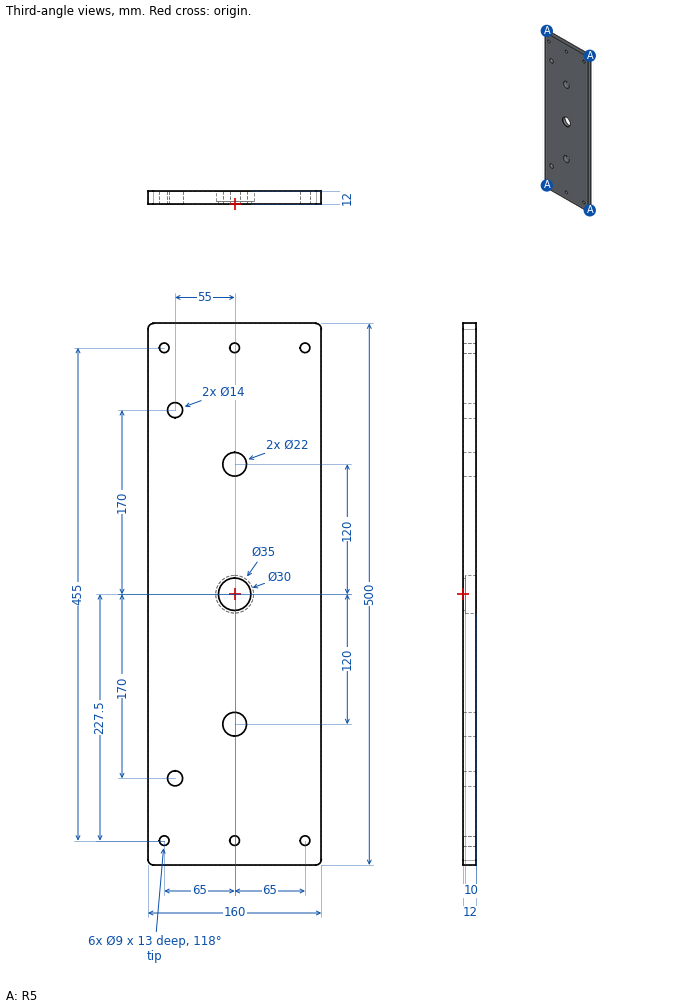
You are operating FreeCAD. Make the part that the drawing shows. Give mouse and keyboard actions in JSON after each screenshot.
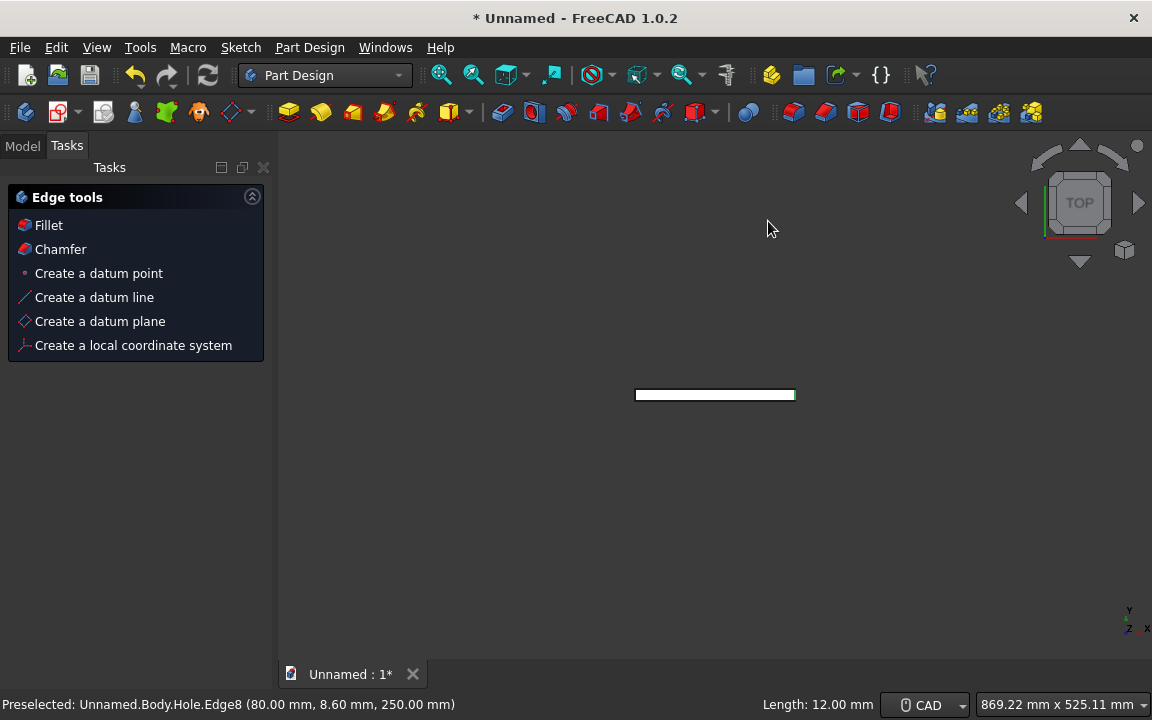
{"action": "left_click", "coordinate": [635, 394], "text": "ctrl"}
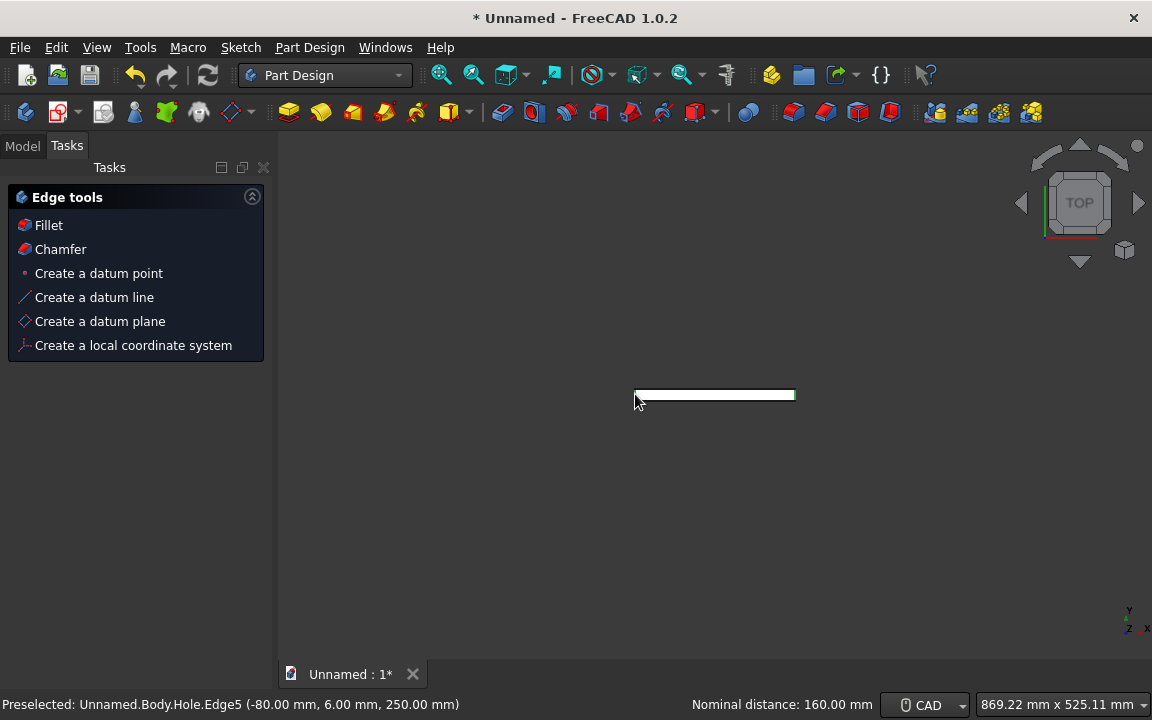
{"action": "scroll", "coordinate": [635, 394], "scroll_direction": "up", "scroll_amount": 6}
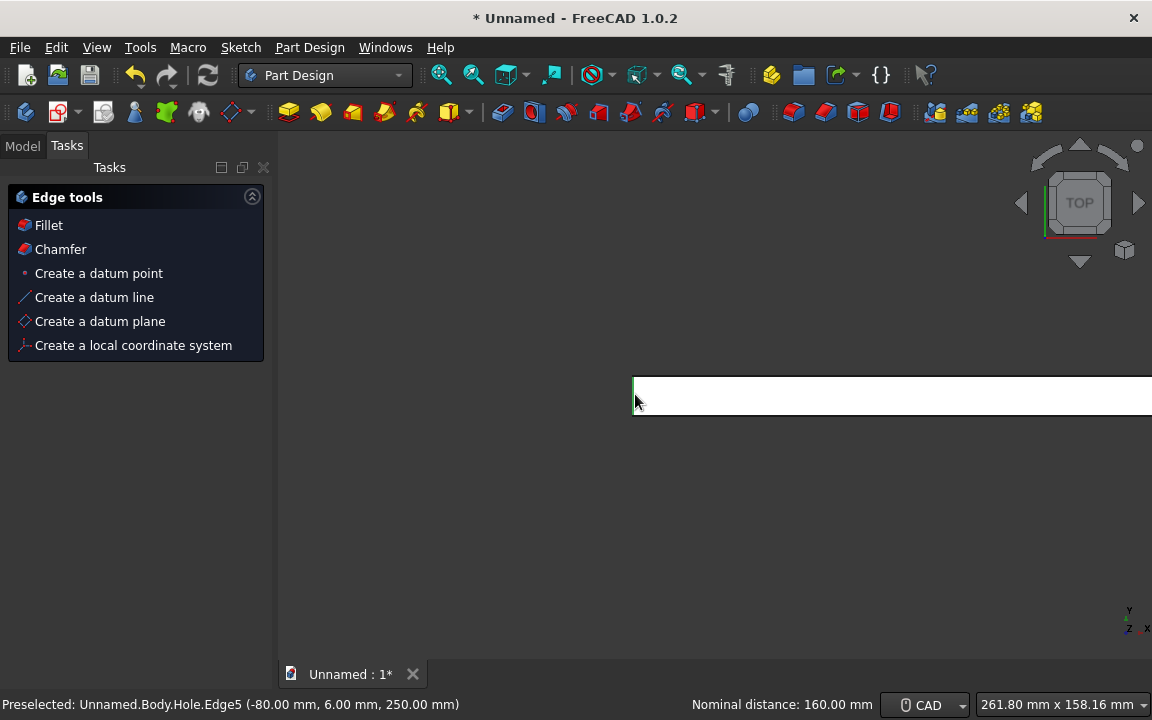
{"action": "key", "text": "v f"}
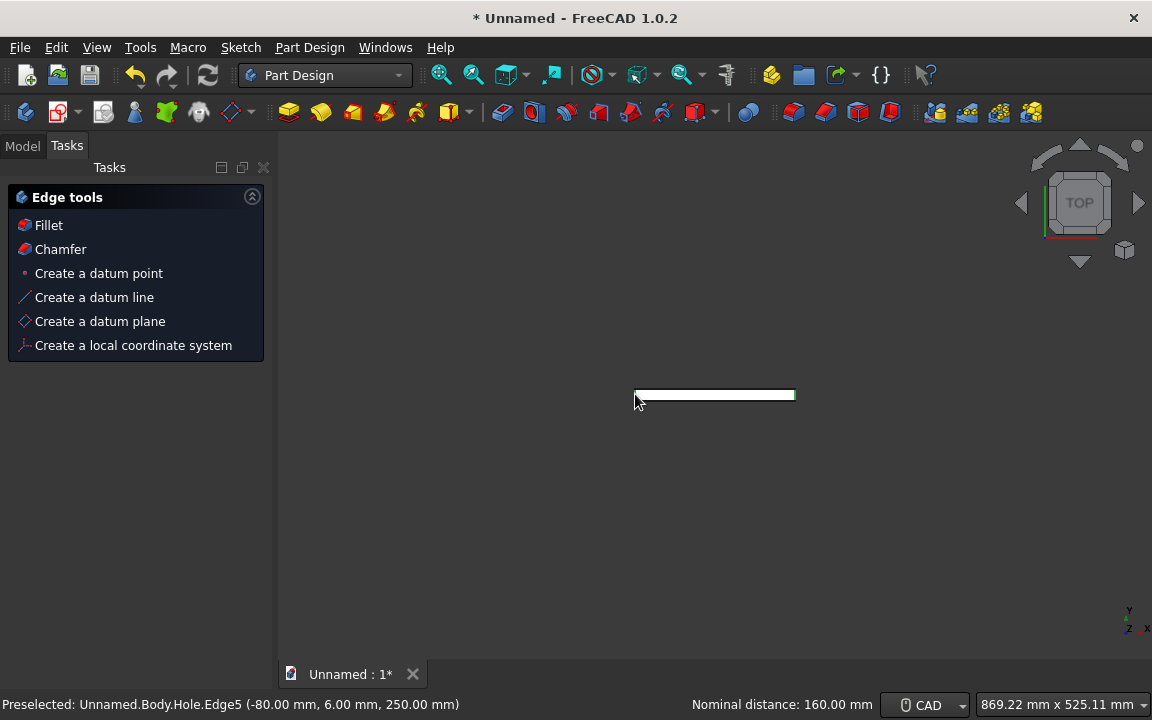
{"action": "key", "text": "1"}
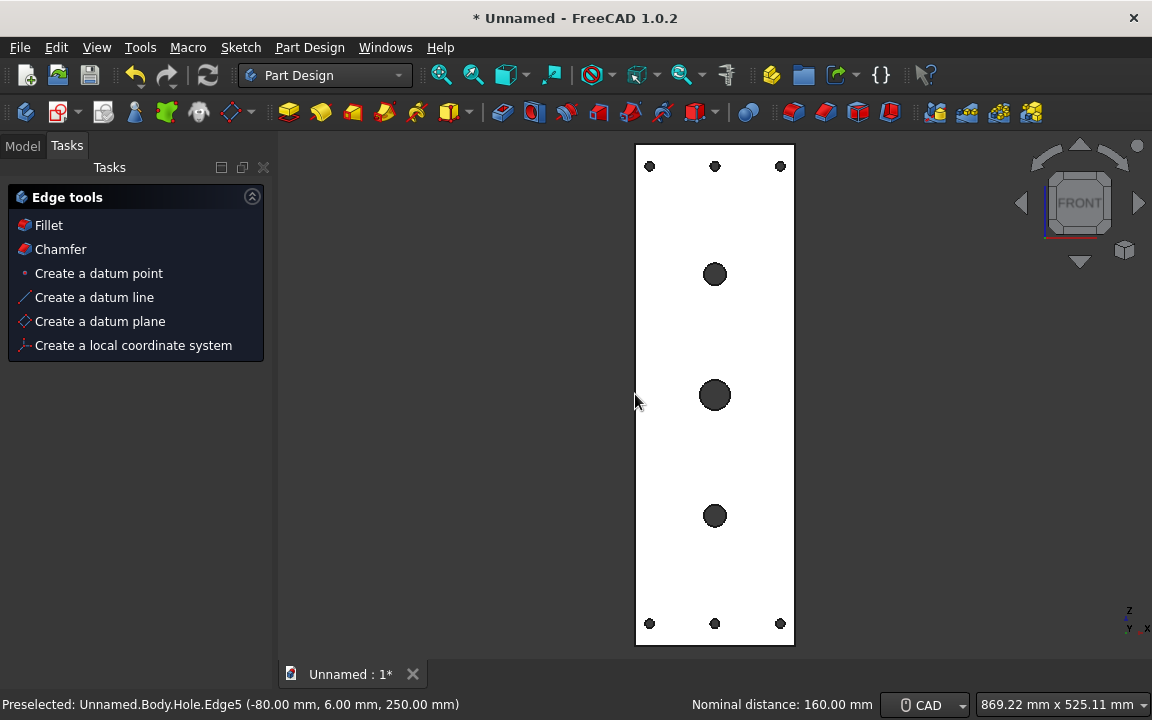
{"action": "key", "text": "3"}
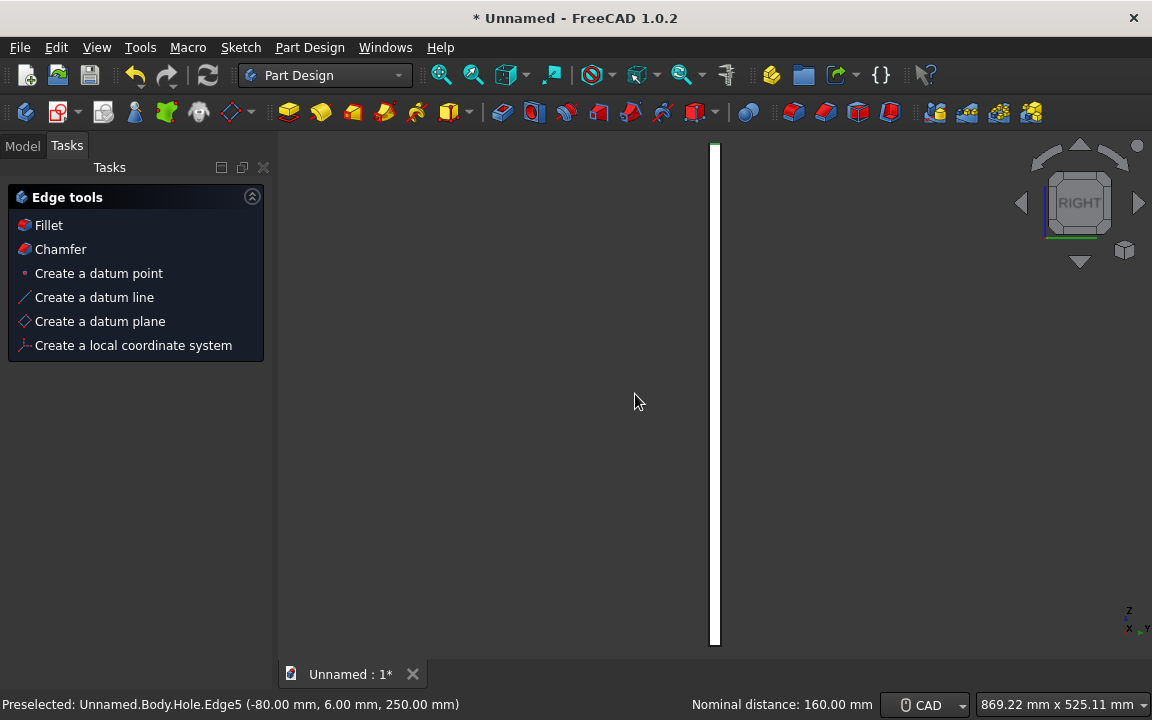
{"action": "key", "text": "5"}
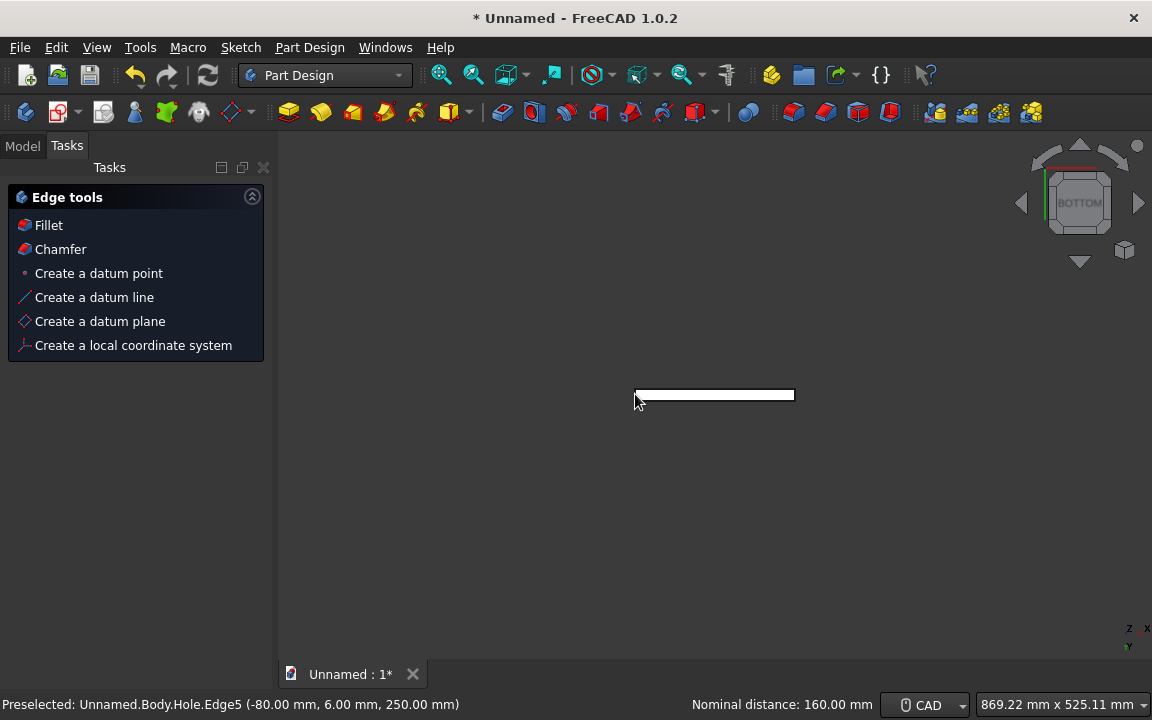
{"action": "left_click", "coordinate": [442, 76]}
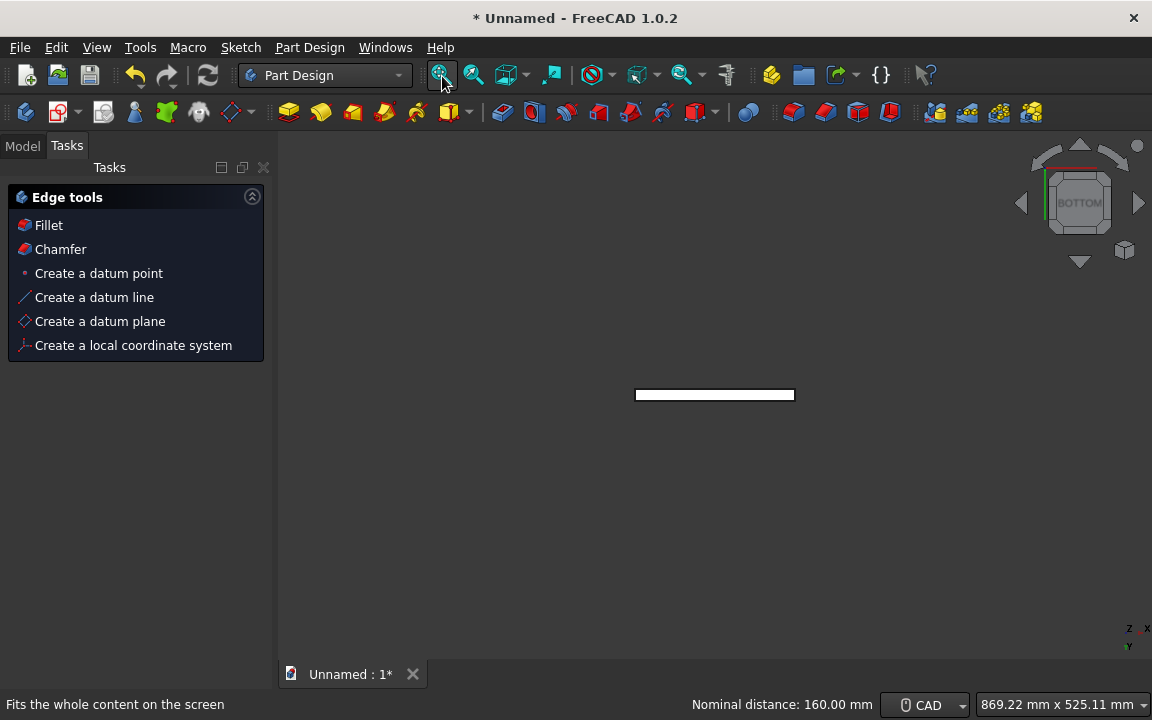
{"action": "left_click", "coordinate": [635, 394], "text": "ctrl"}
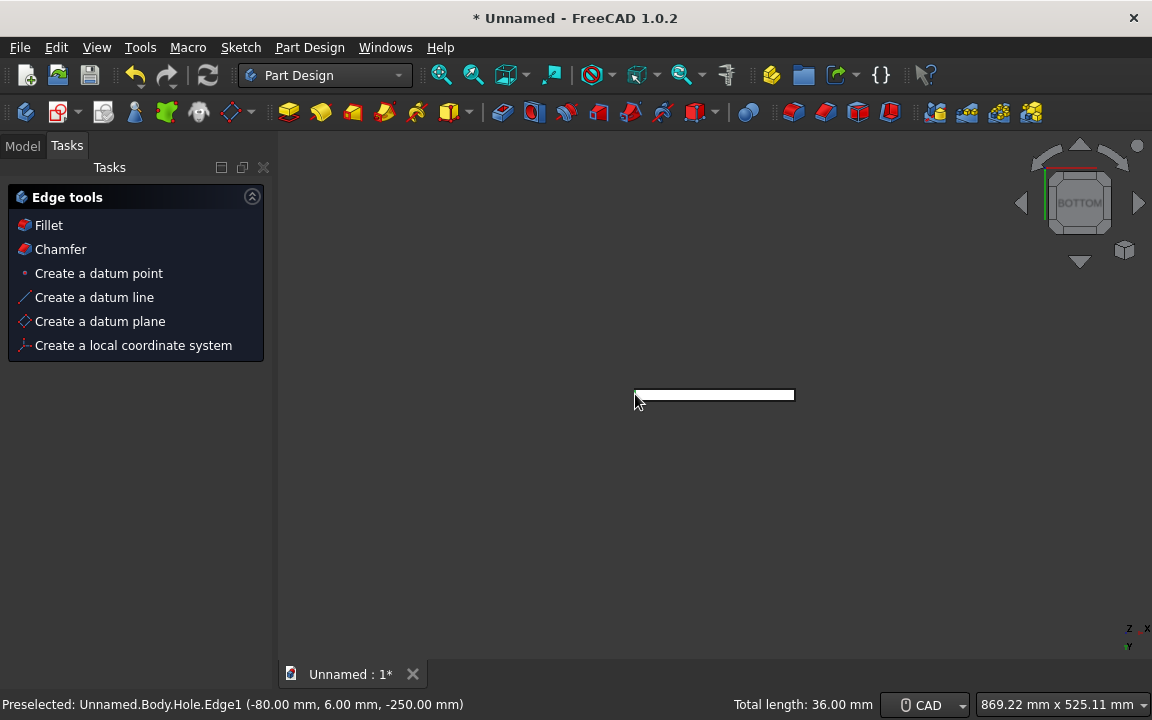
{"action": "left_click", "coordinate": [795, 394], "text": "ctrl"}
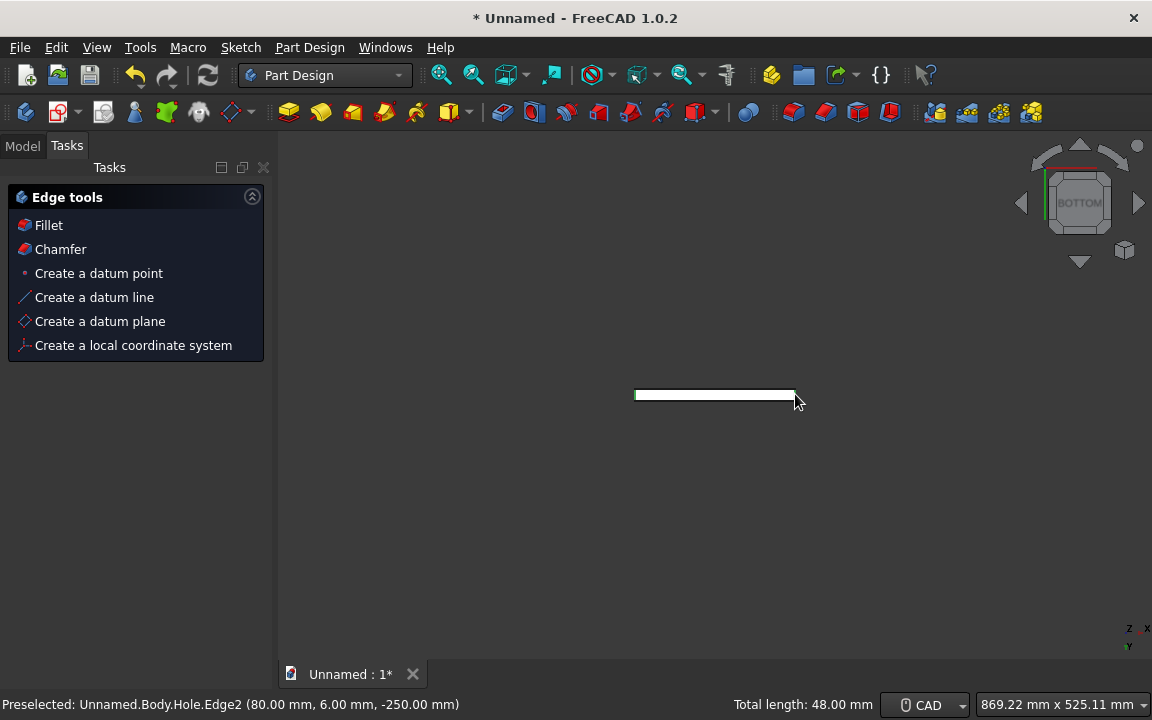
{"action": "left_click", "coordinate": [794, 112]}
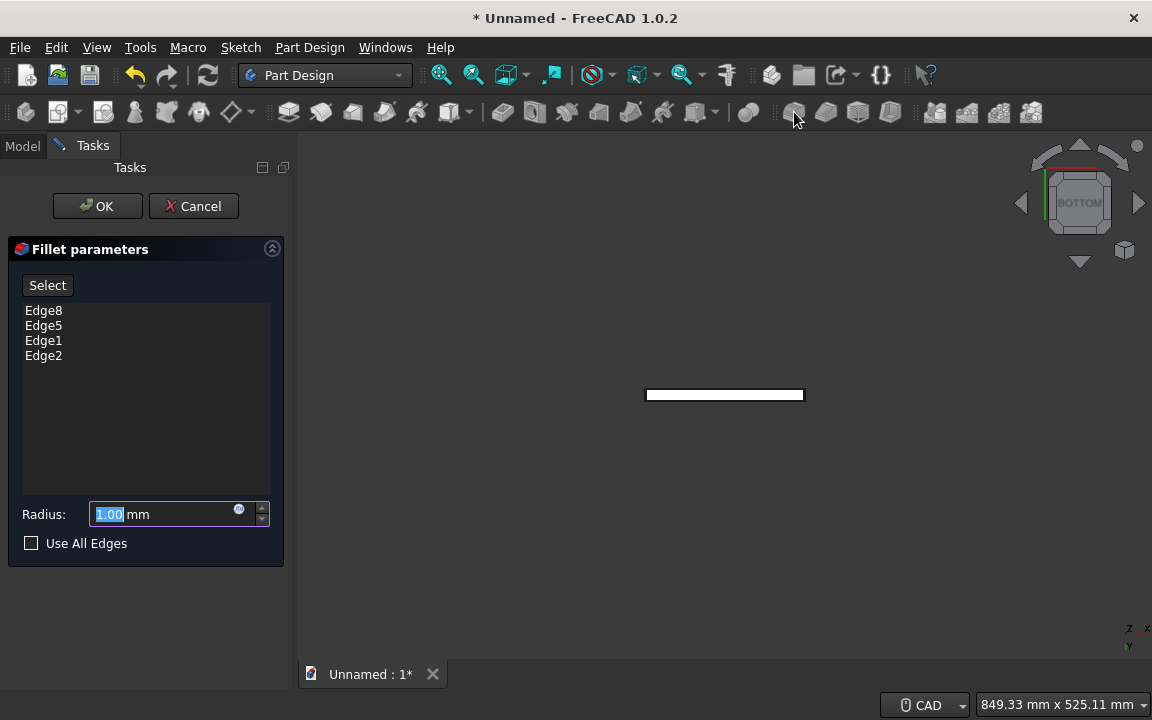
{"action": "type", "text": "5"}
{"action": "key", "text": "Tab"}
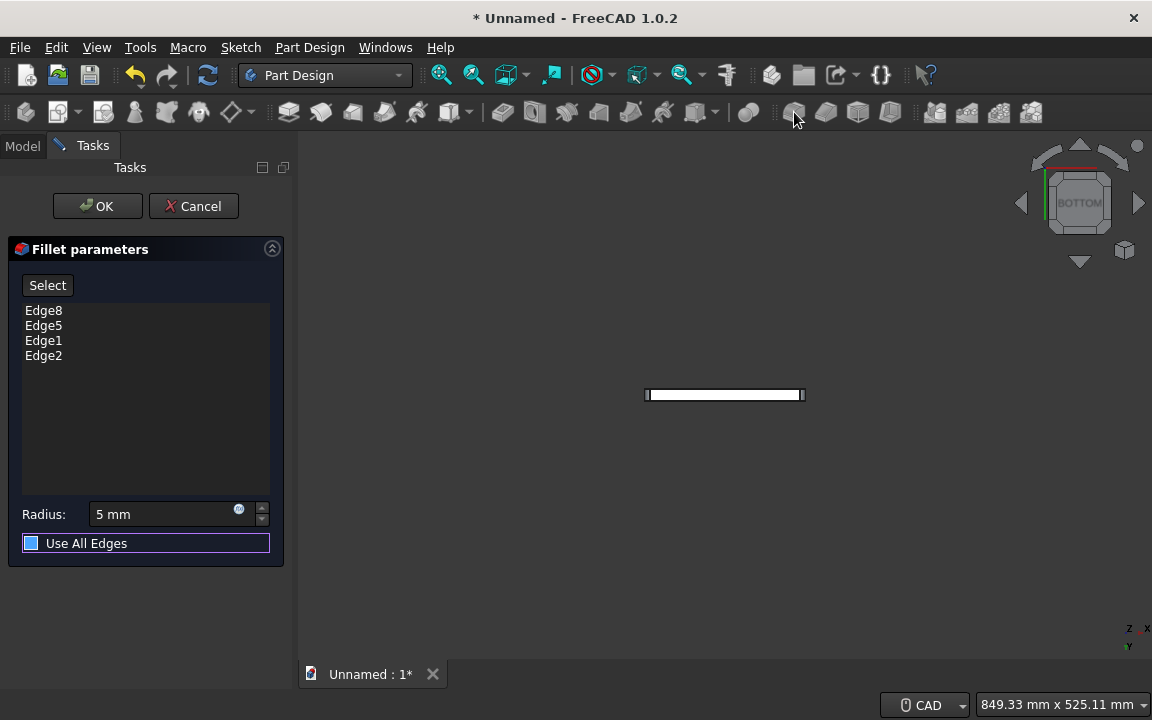
{"action": "left_click", "coordinate": [98, 206]}